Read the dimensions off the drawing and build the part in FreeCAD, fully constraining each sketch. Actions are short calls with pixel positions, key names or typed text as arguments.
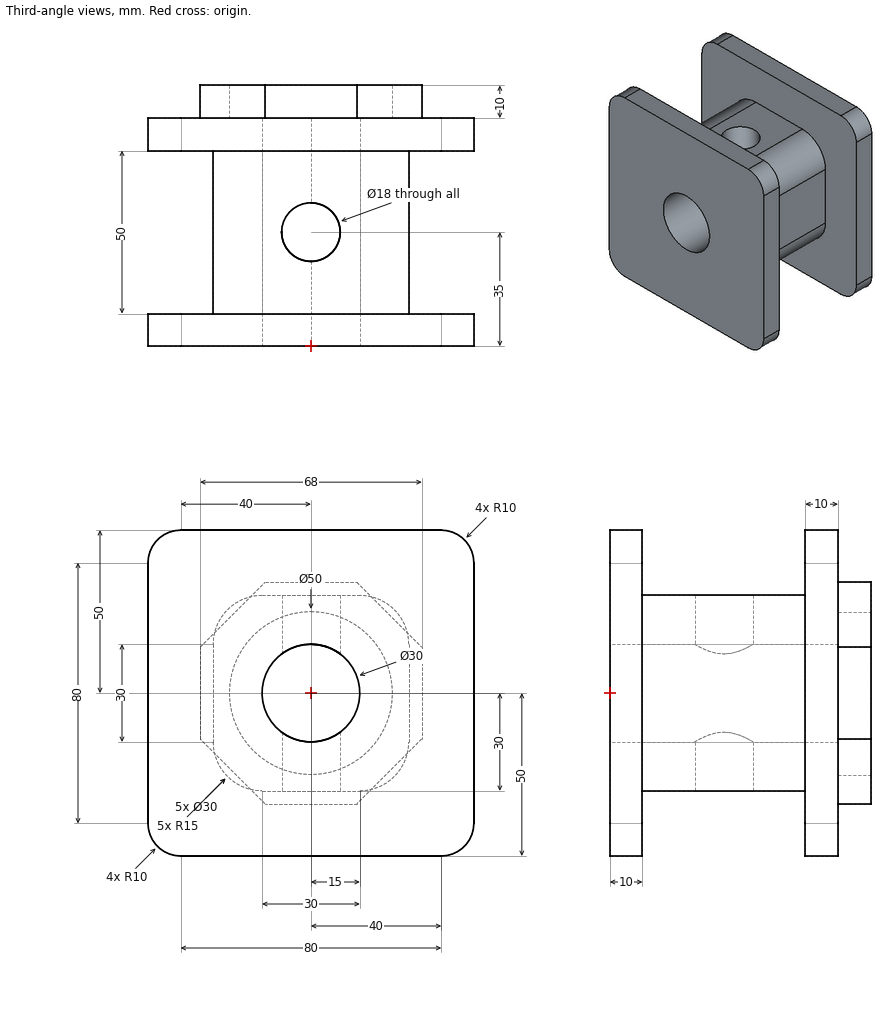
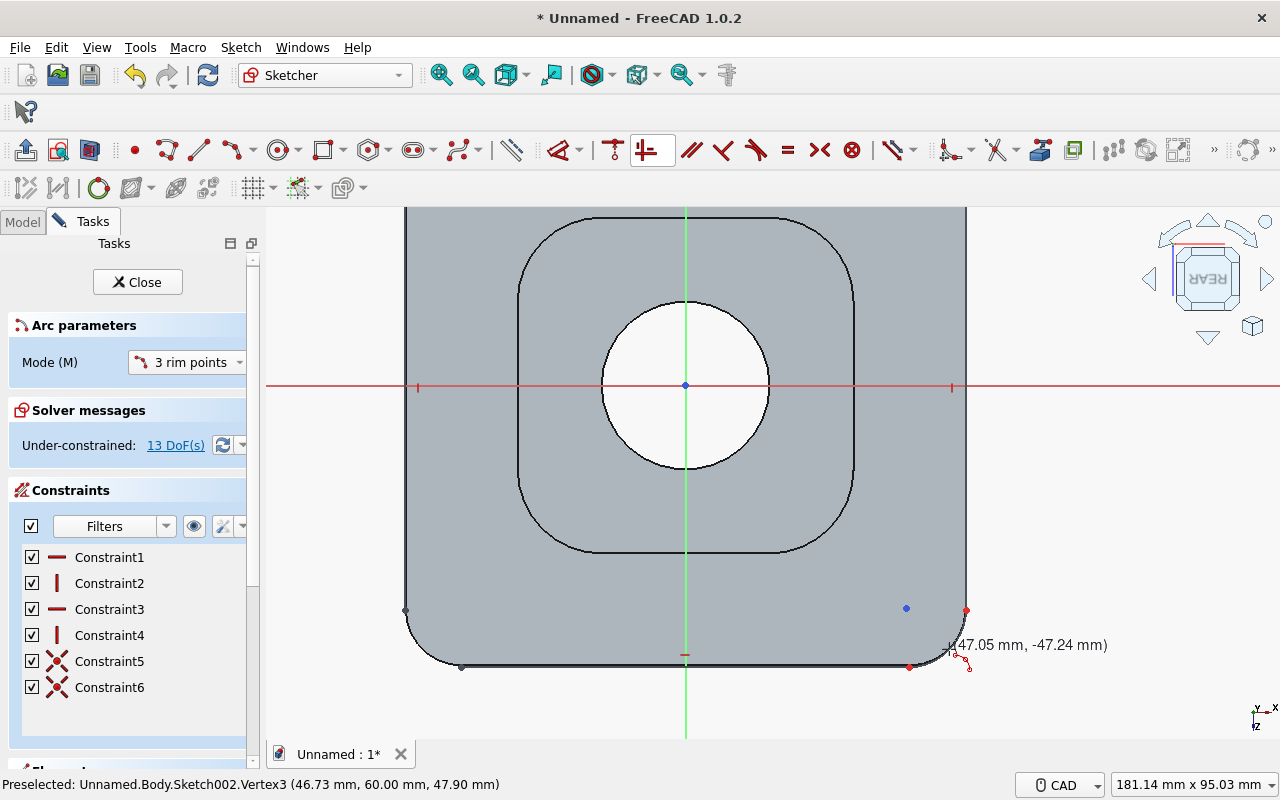
scroll(727, 579, down, 3)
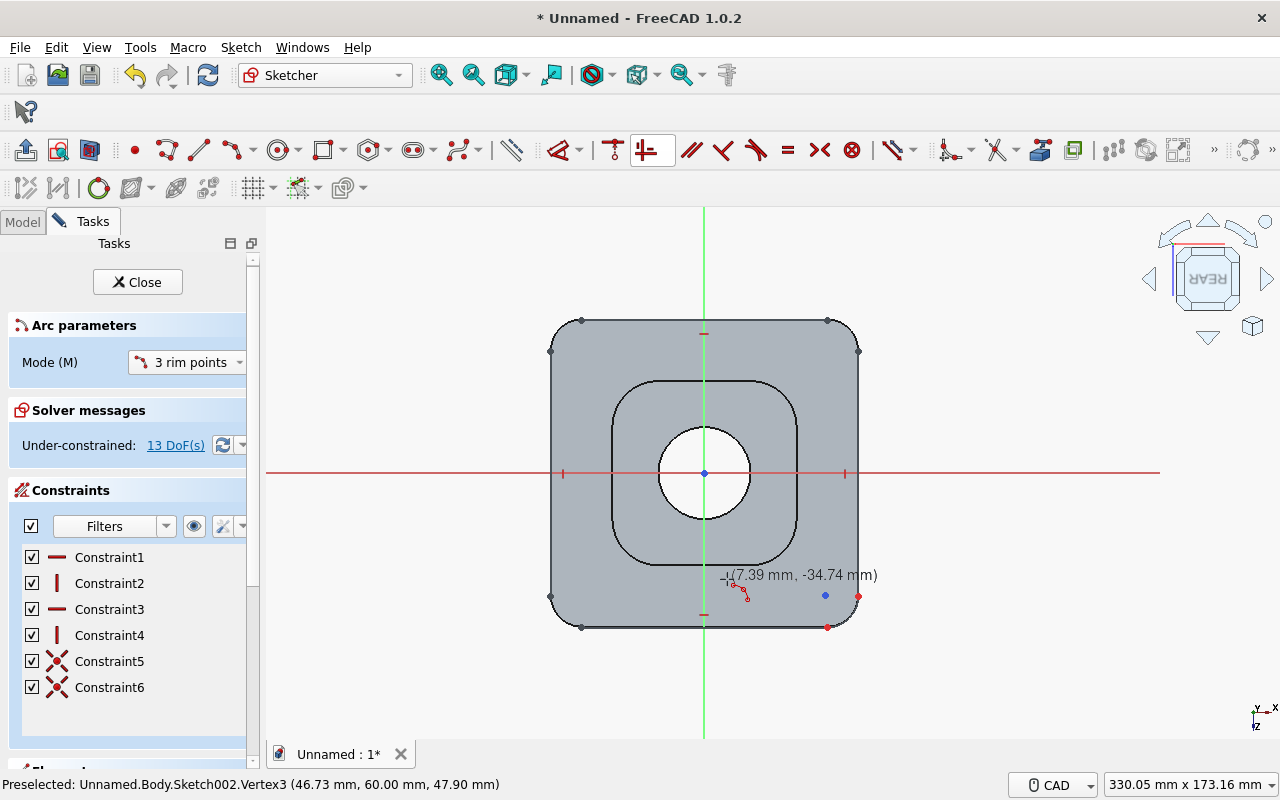
click(858, 351)
click(827, 320)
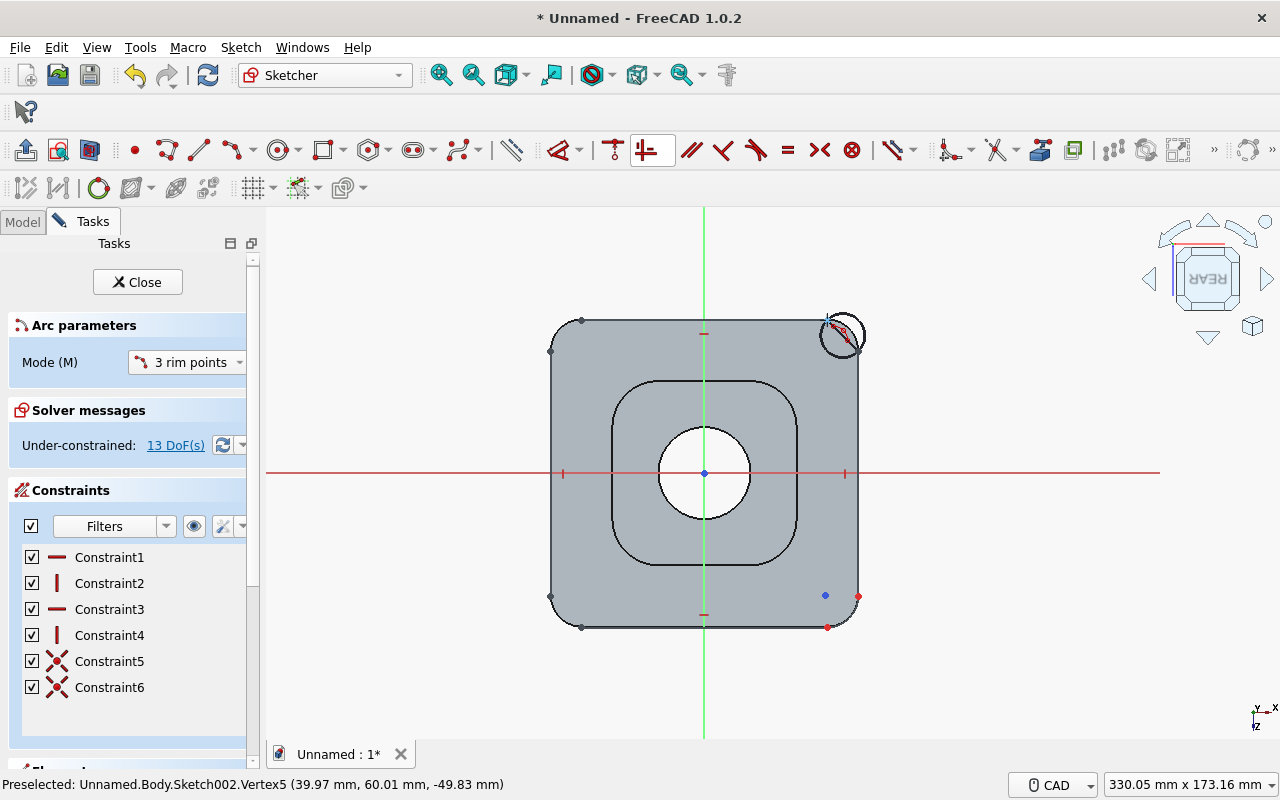
scroll(849, 329, up, 3)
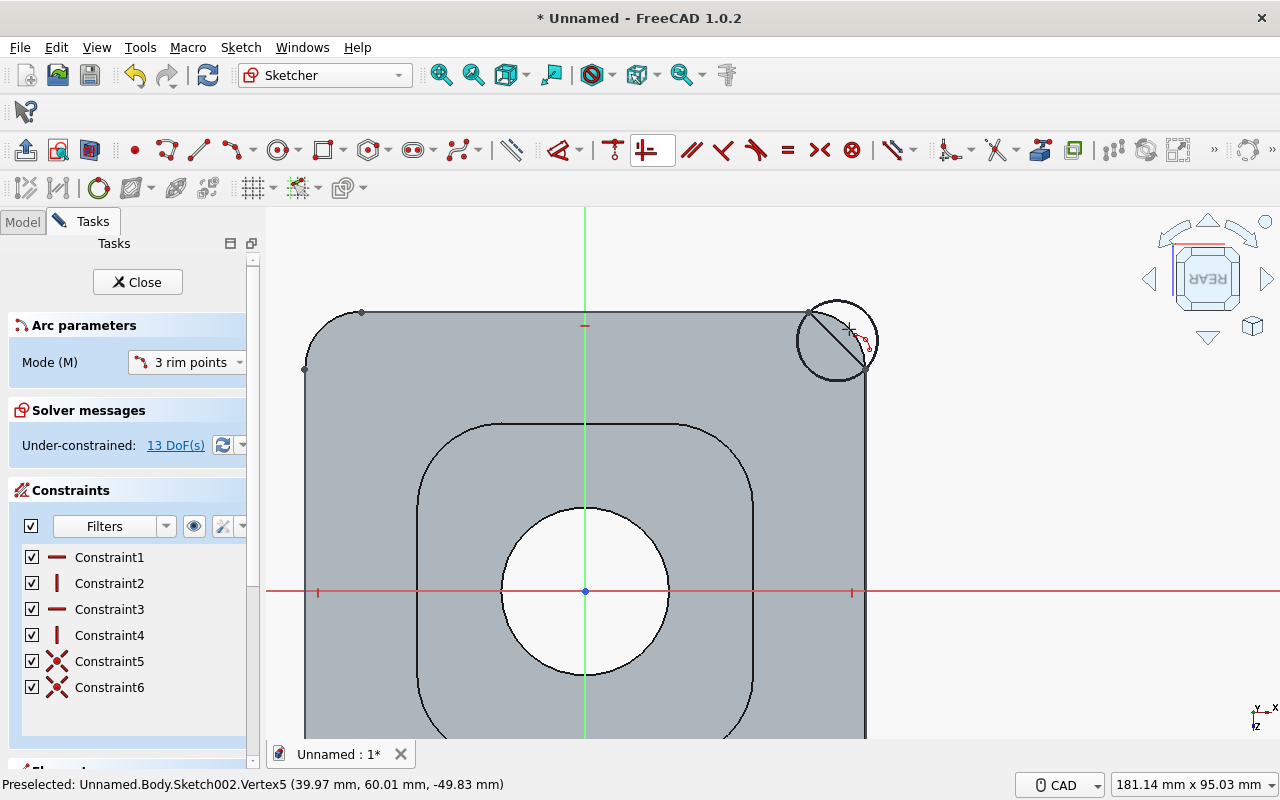
click(849, 328)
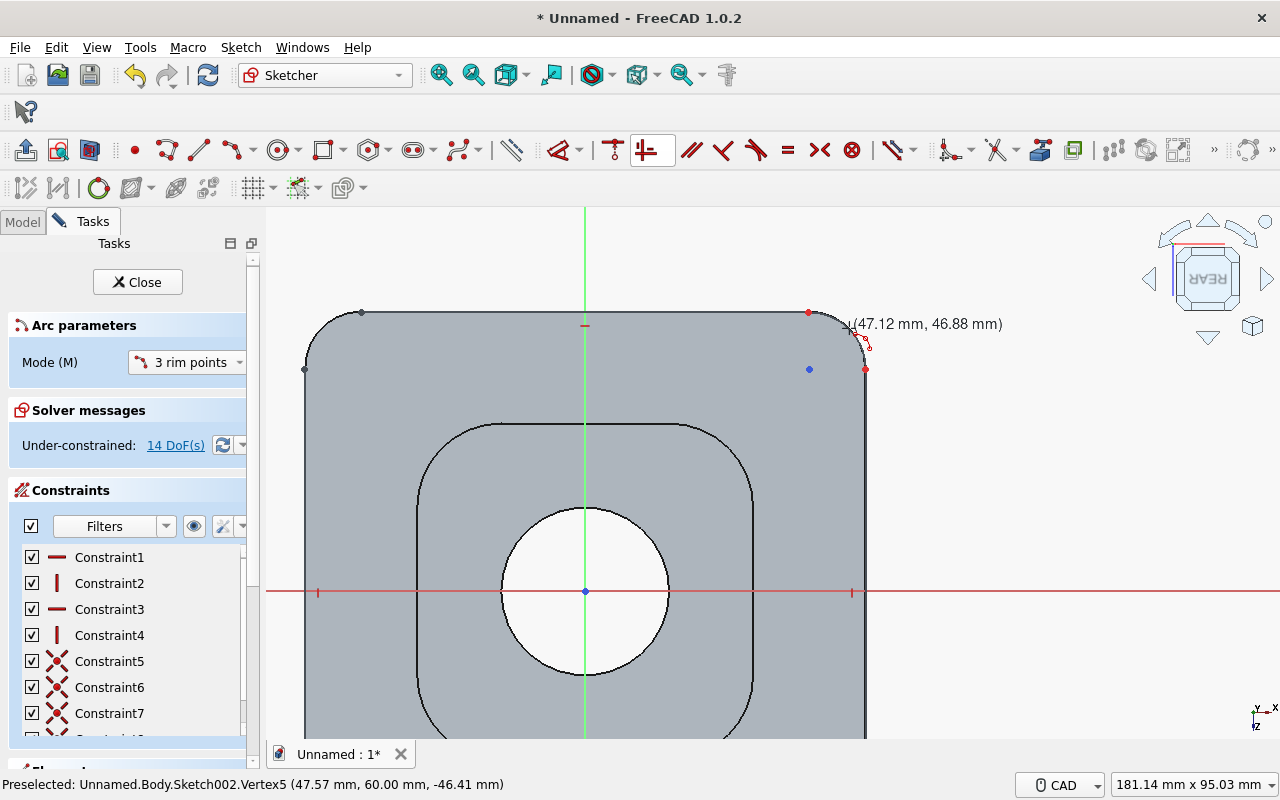
click(361, 312)
click(305, 369)
click(322, 328)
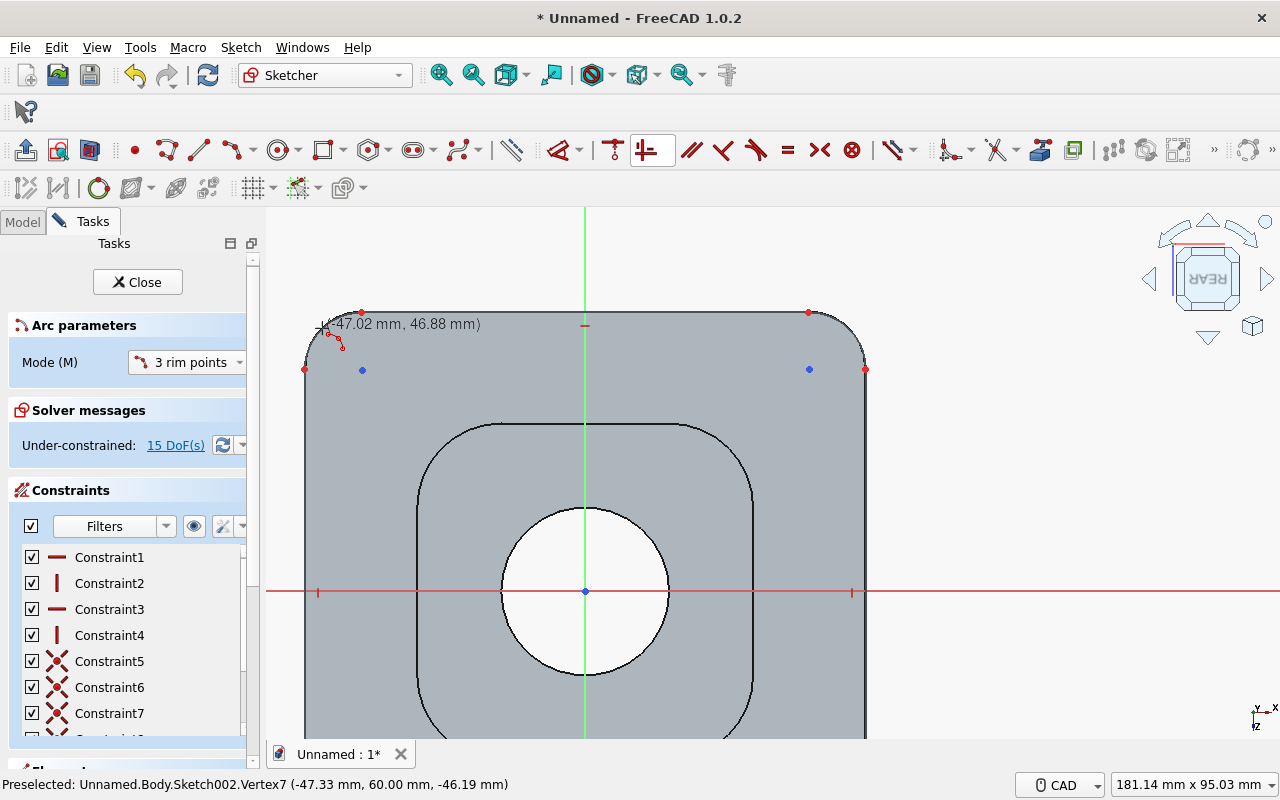
scroll(850, 329, down, 3)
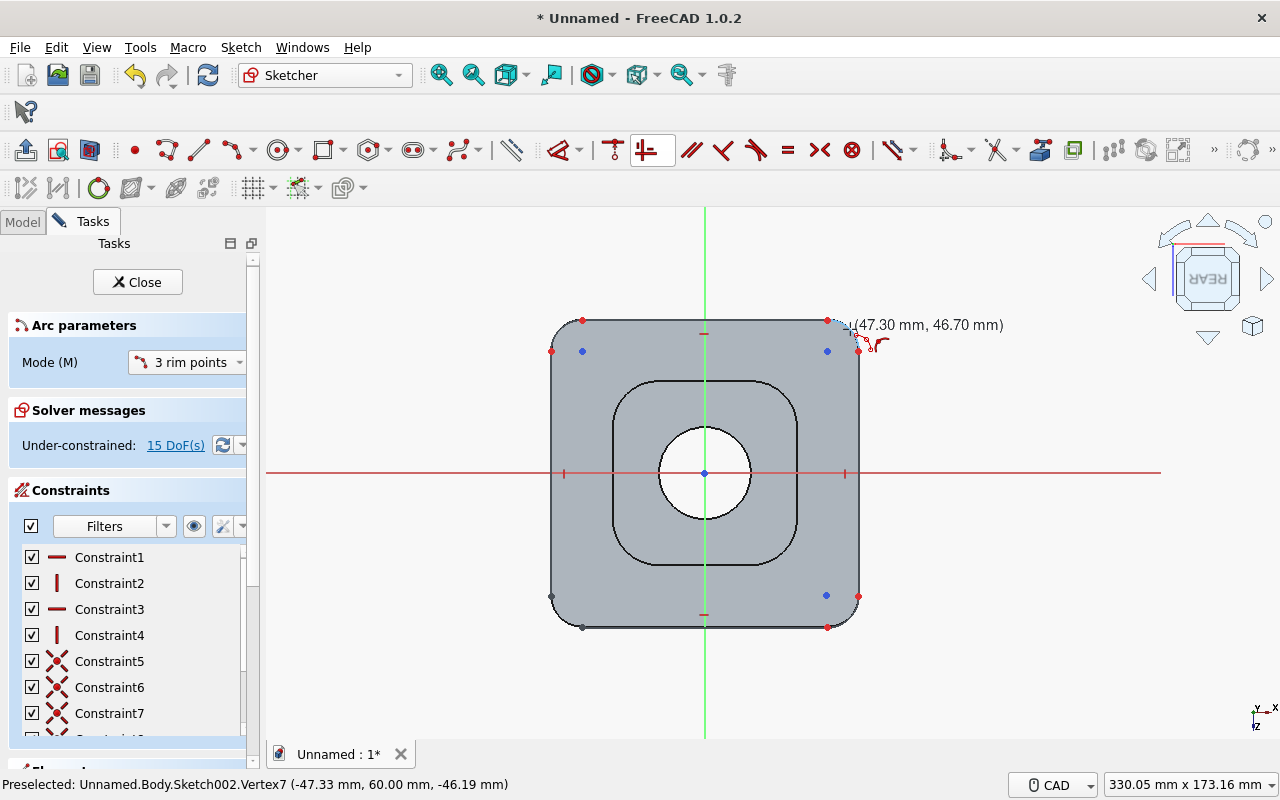
click(551, 597)
click(582, 628)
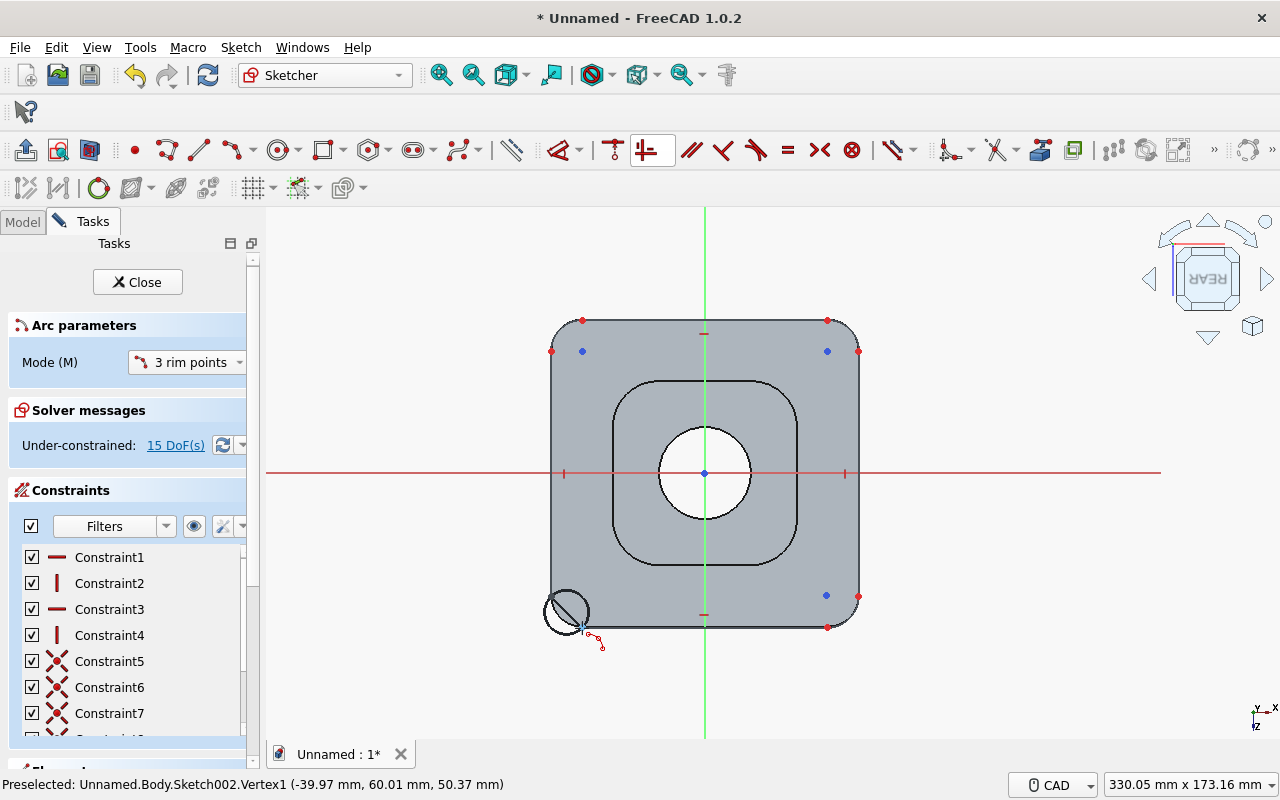
scroll(560, 618, up, 3)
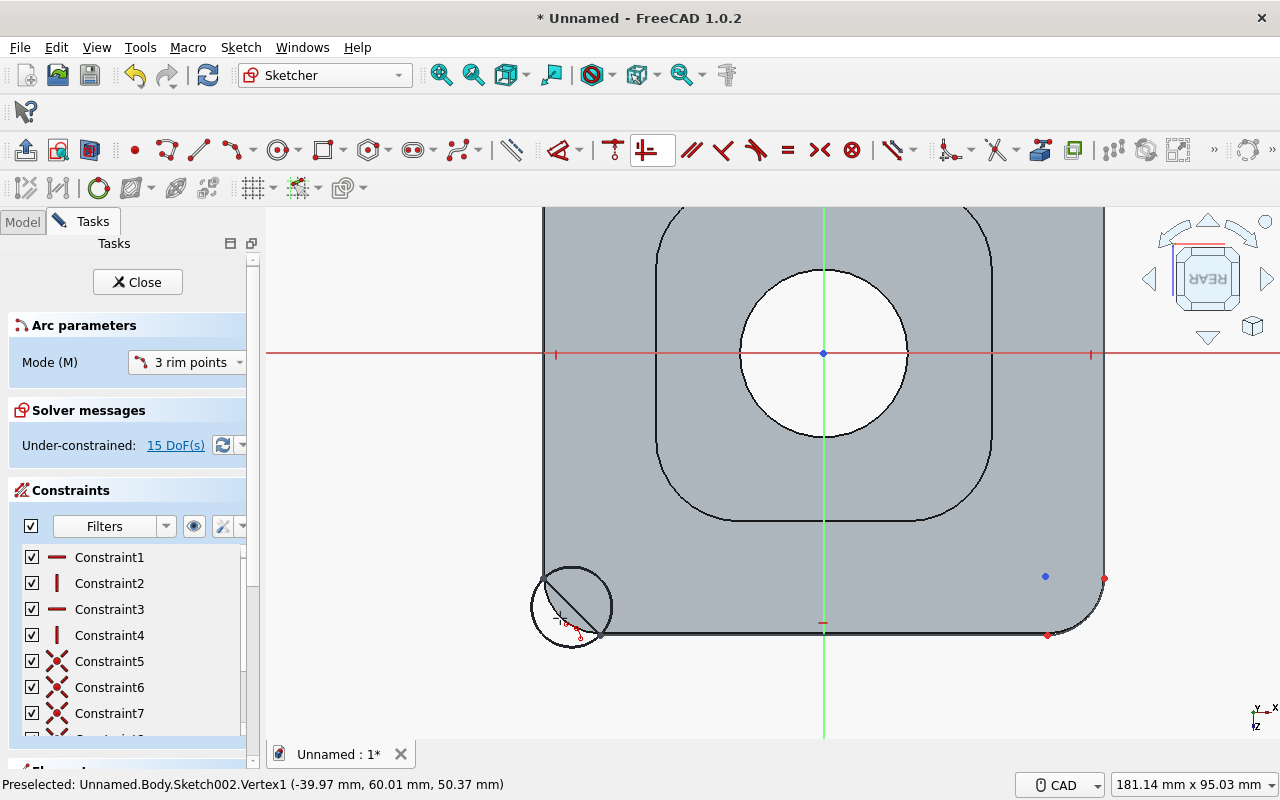
click(560, 617)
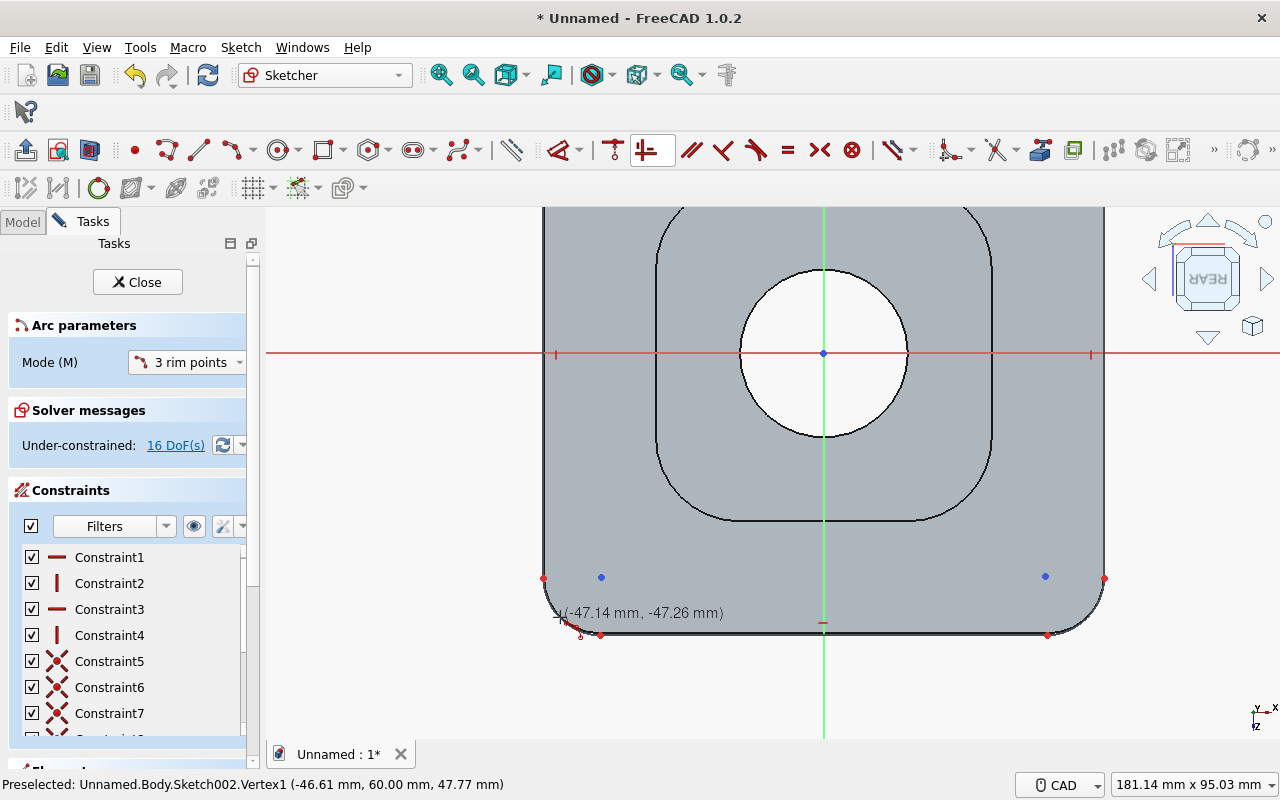
click(278, 150)